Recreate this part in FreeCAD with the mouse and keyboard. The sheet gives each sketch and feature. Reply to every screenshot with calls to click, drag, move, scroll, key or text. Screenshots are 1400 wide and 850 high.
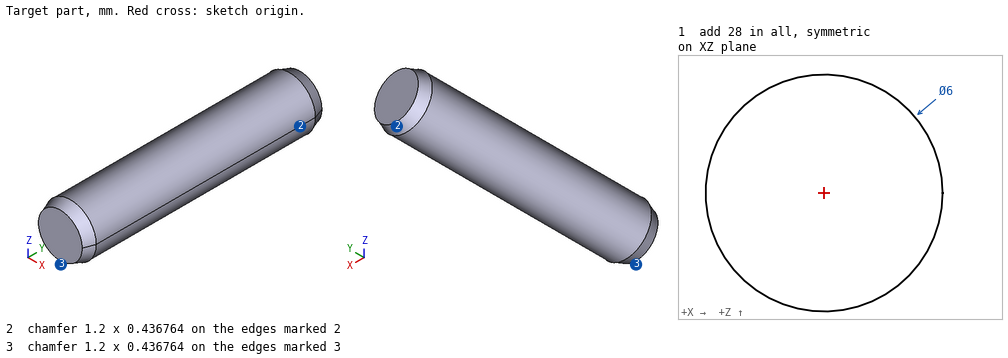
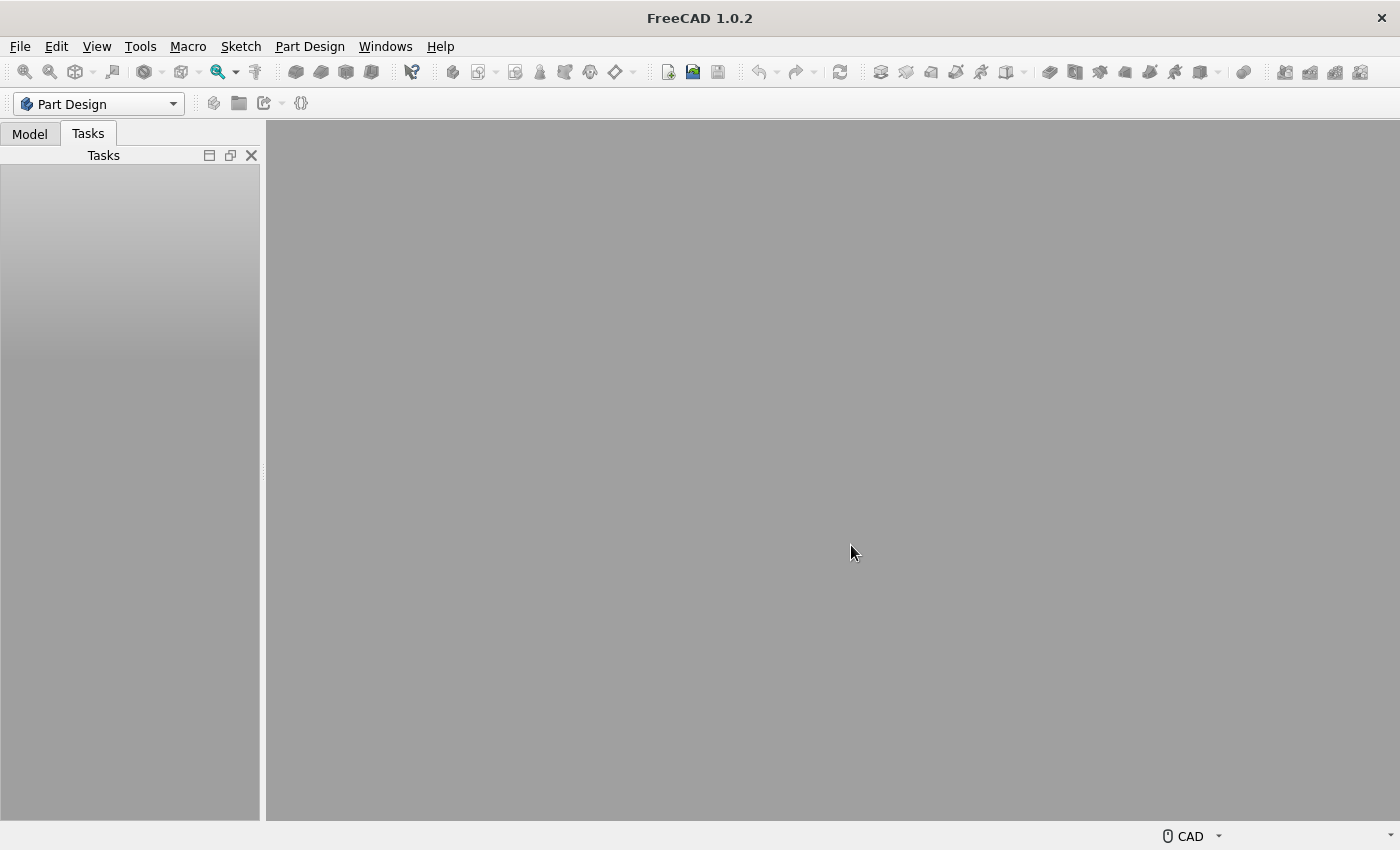
key(ctrl+n)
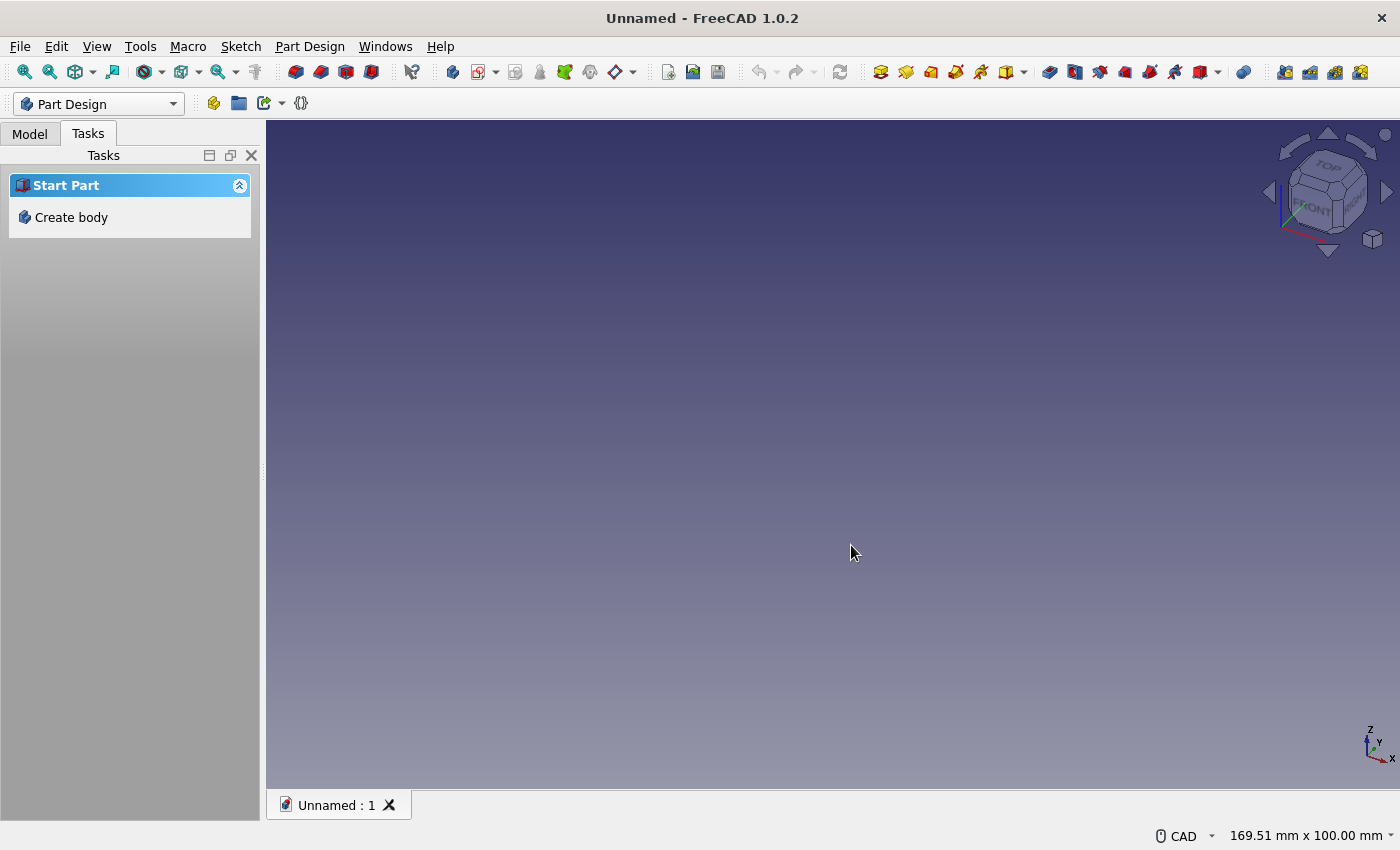
click(478, 72)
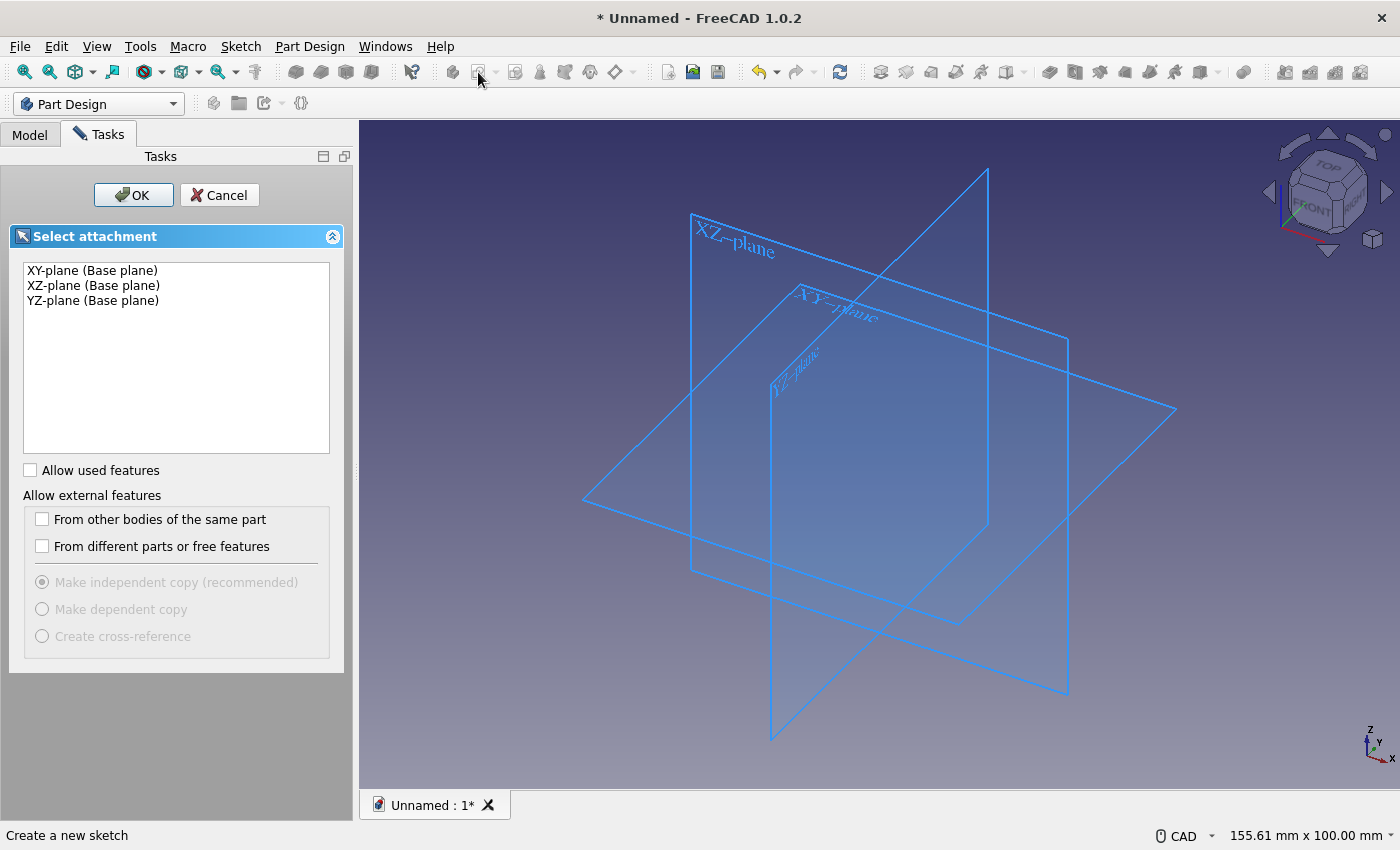
click(84, 286)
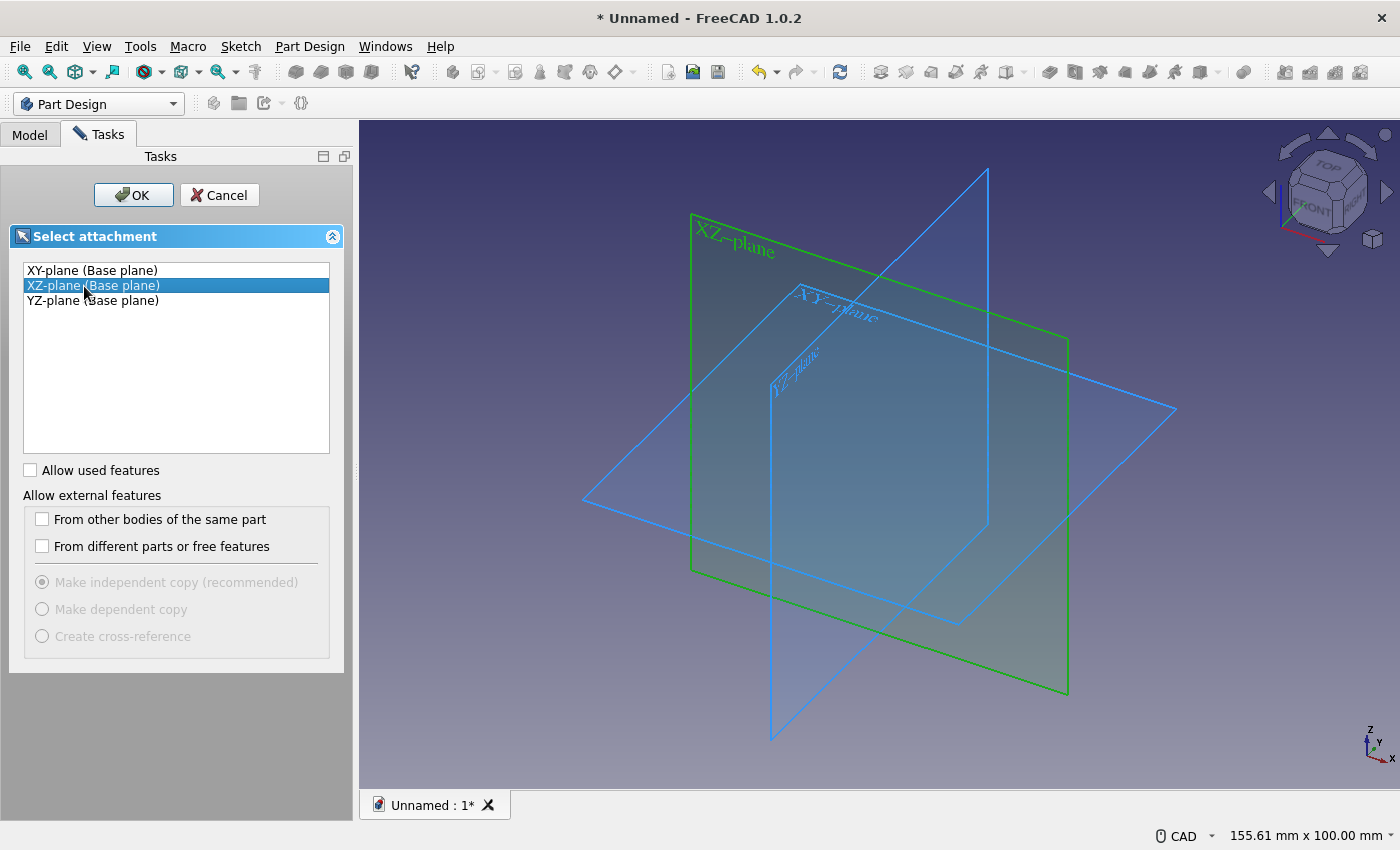
click(134, 195)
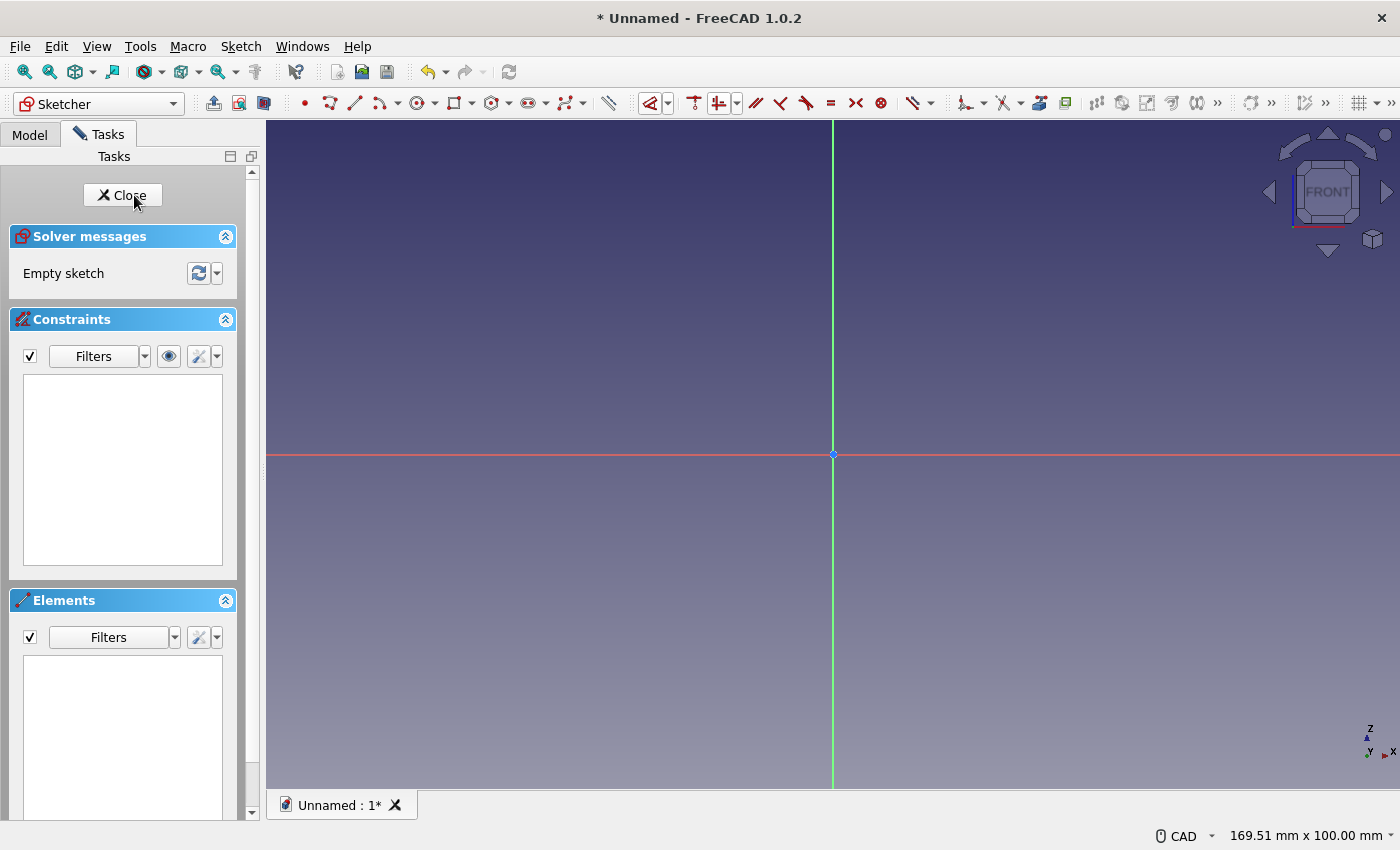
scroll(840, 455, up, 12)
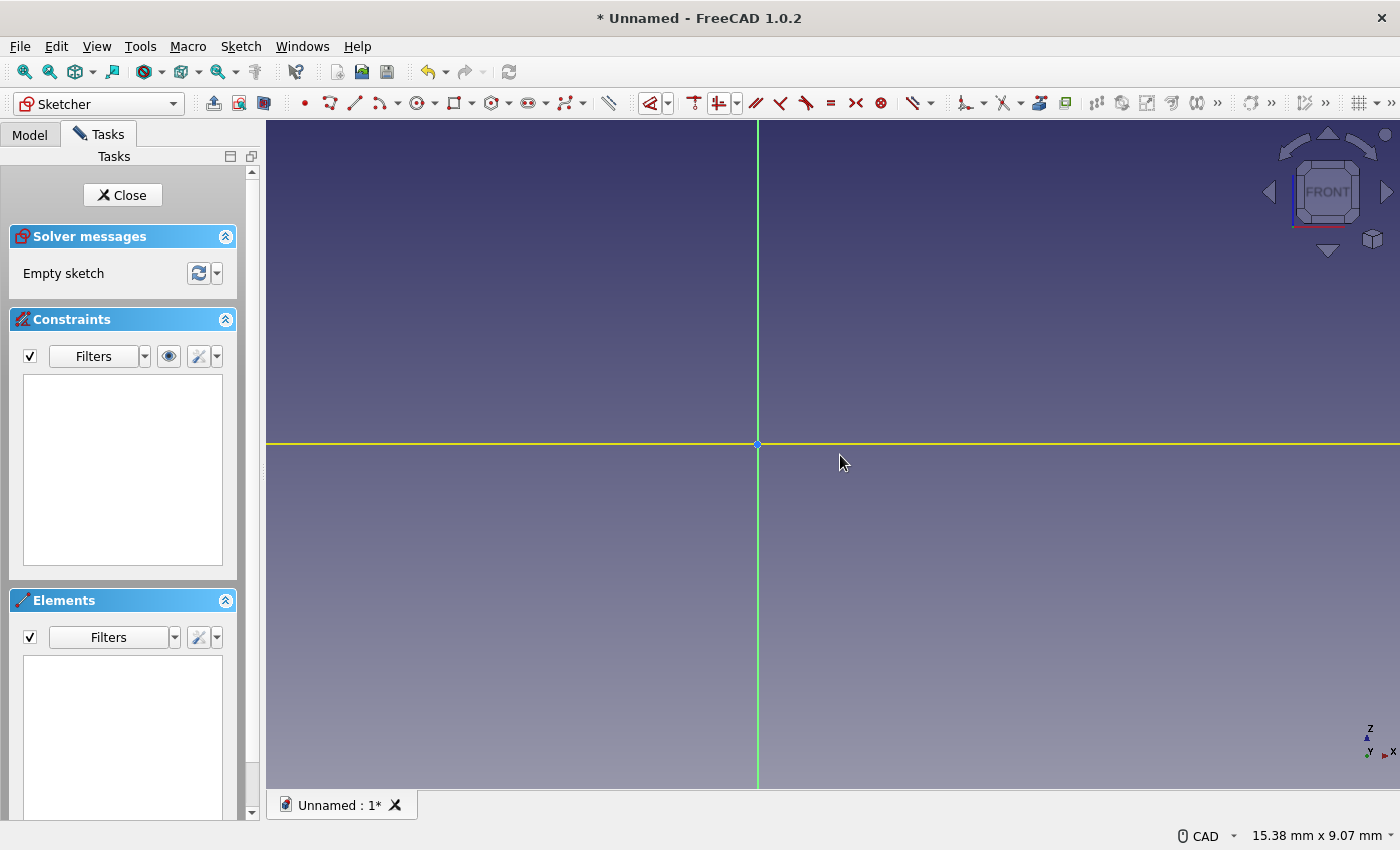
click(416, 104)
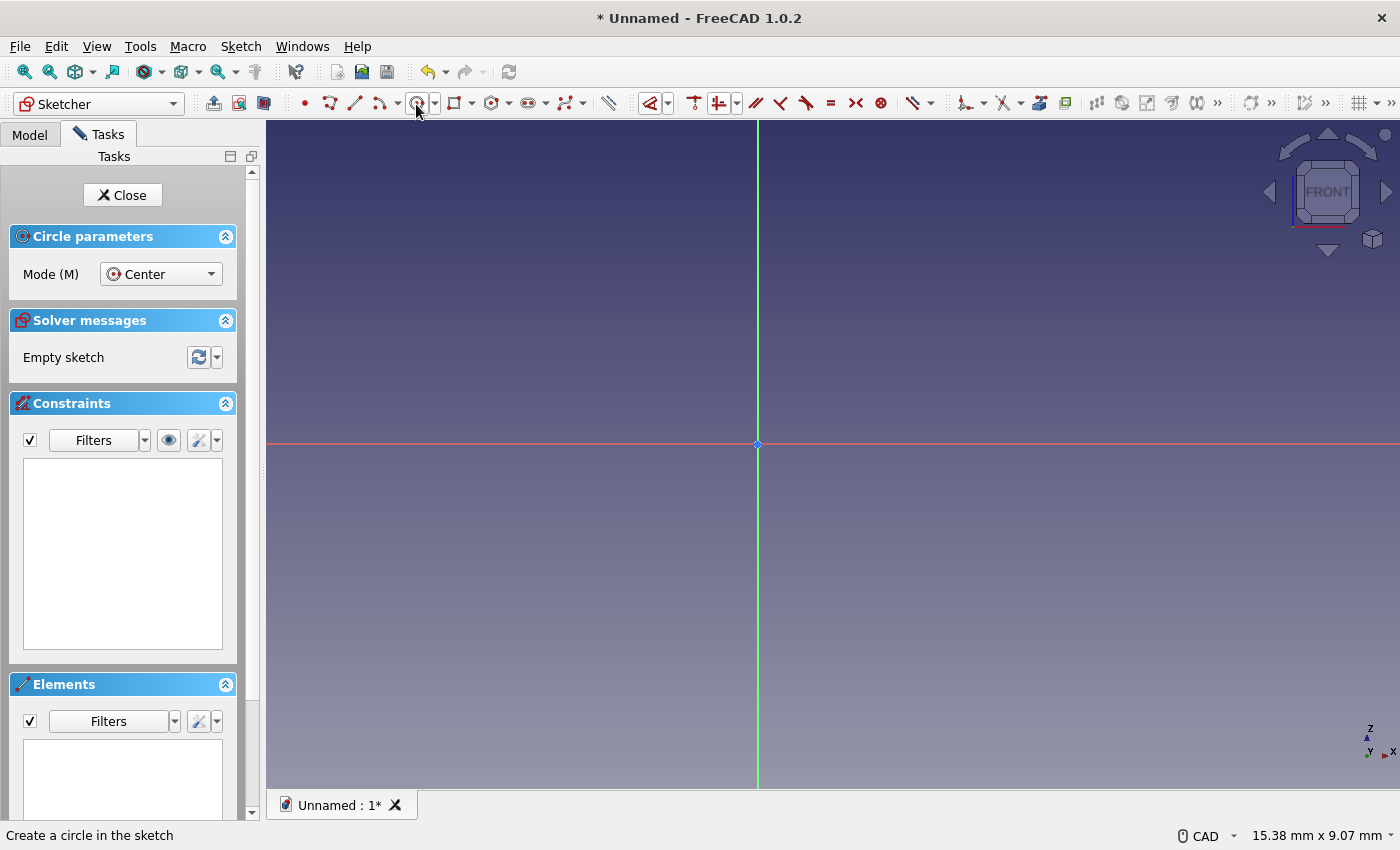
click(758, 444)
click(914, 288)
key(Escape)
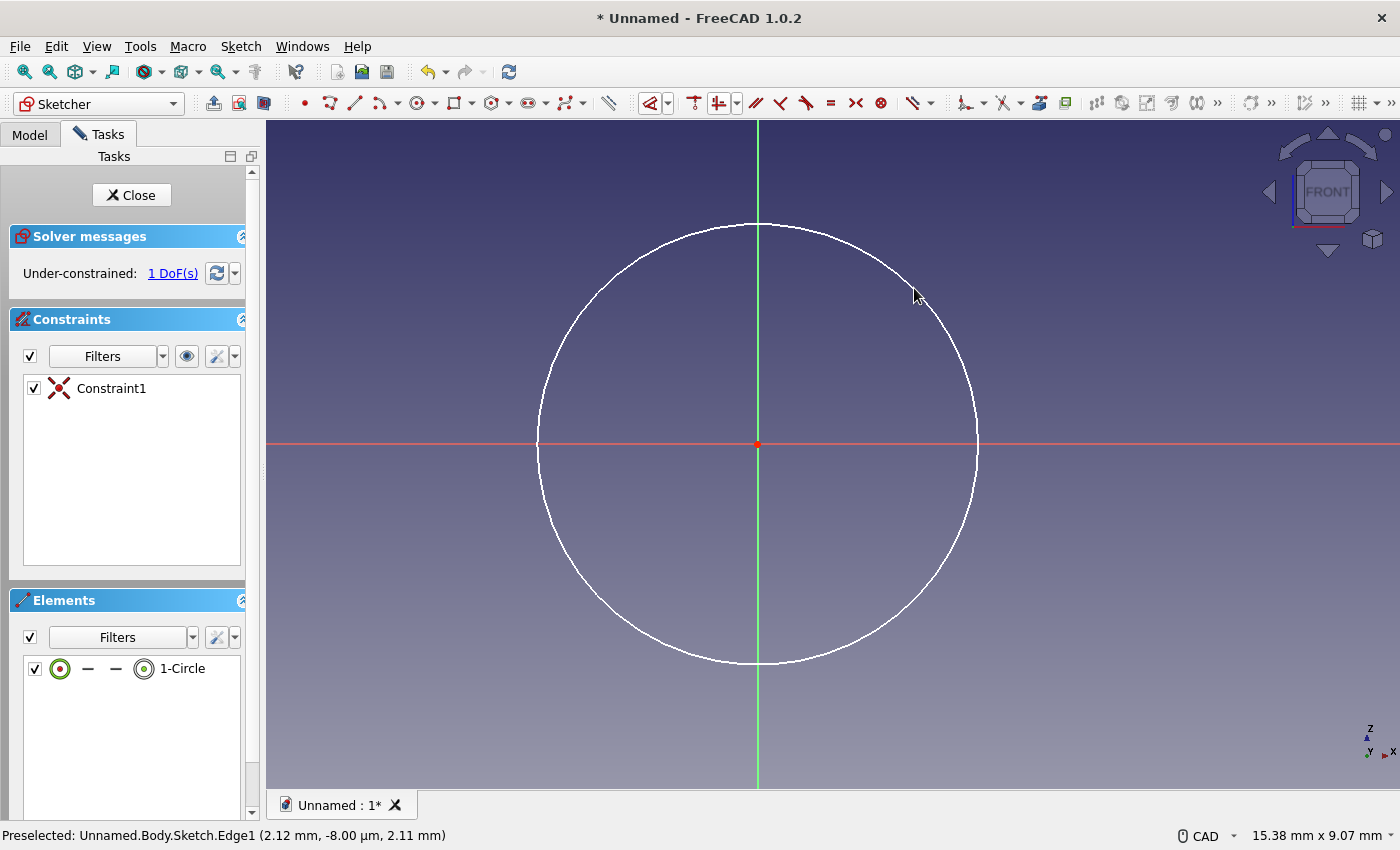
key(d)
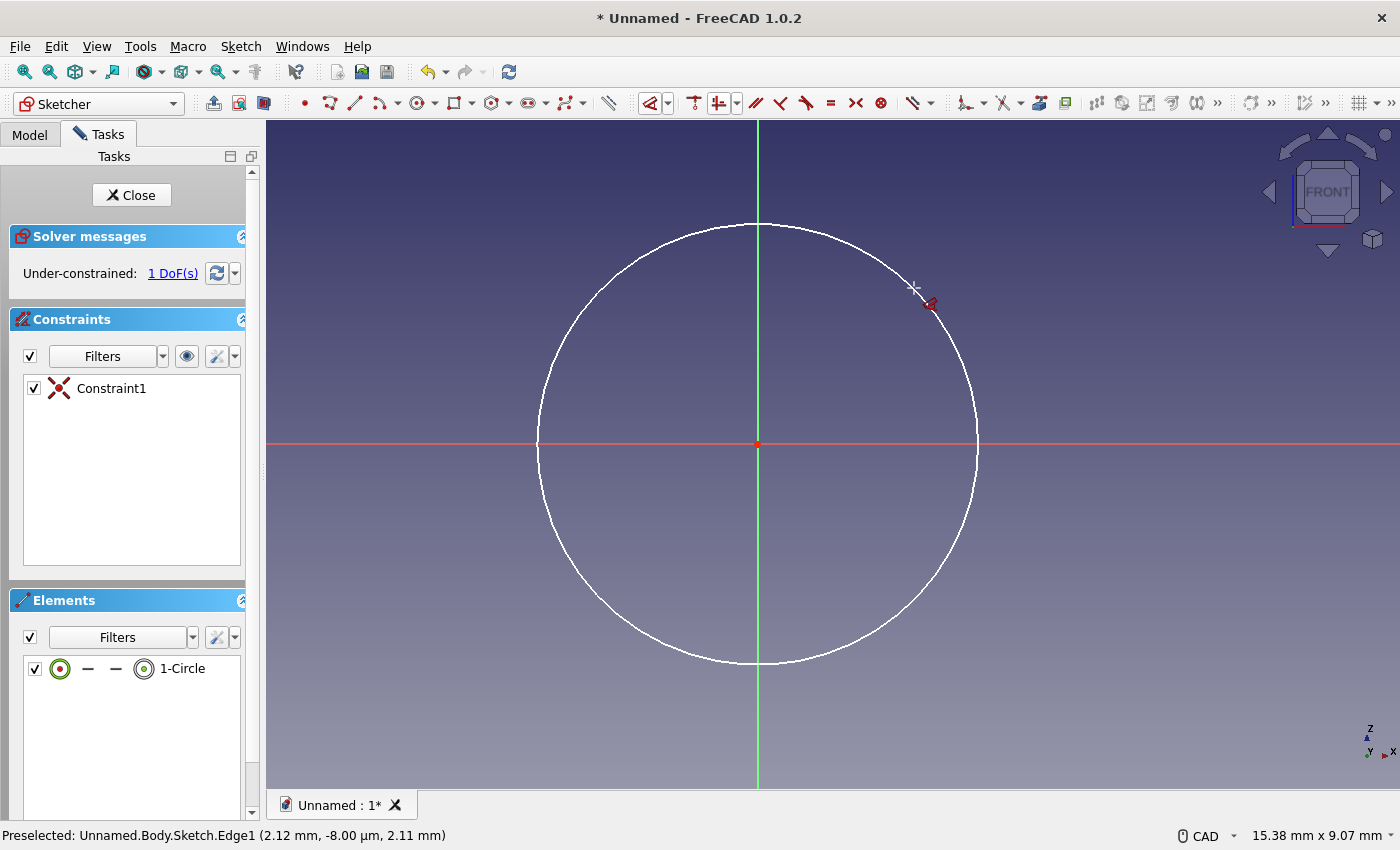
click(913, 288)
click(936, 265)